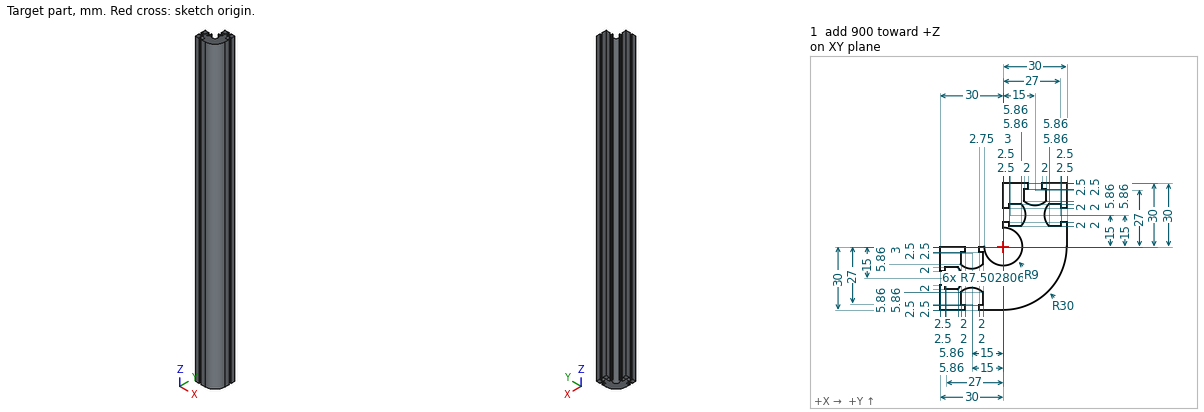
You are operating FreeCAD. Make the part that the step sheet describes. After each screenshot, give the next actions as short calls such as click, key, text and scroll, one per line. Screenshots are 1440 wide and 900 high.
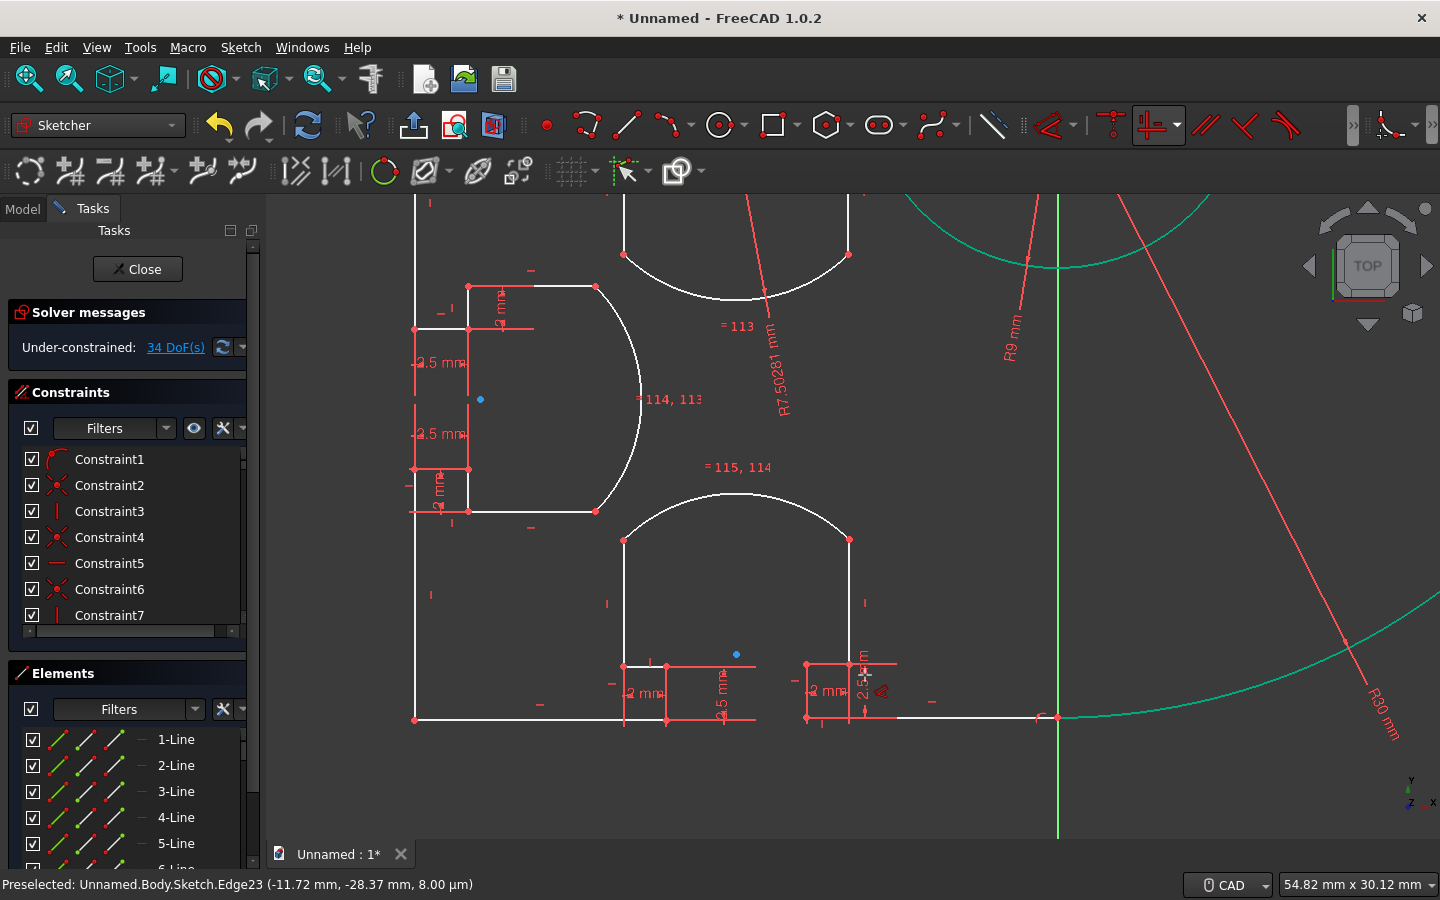
scroll(667, 707, down, 6)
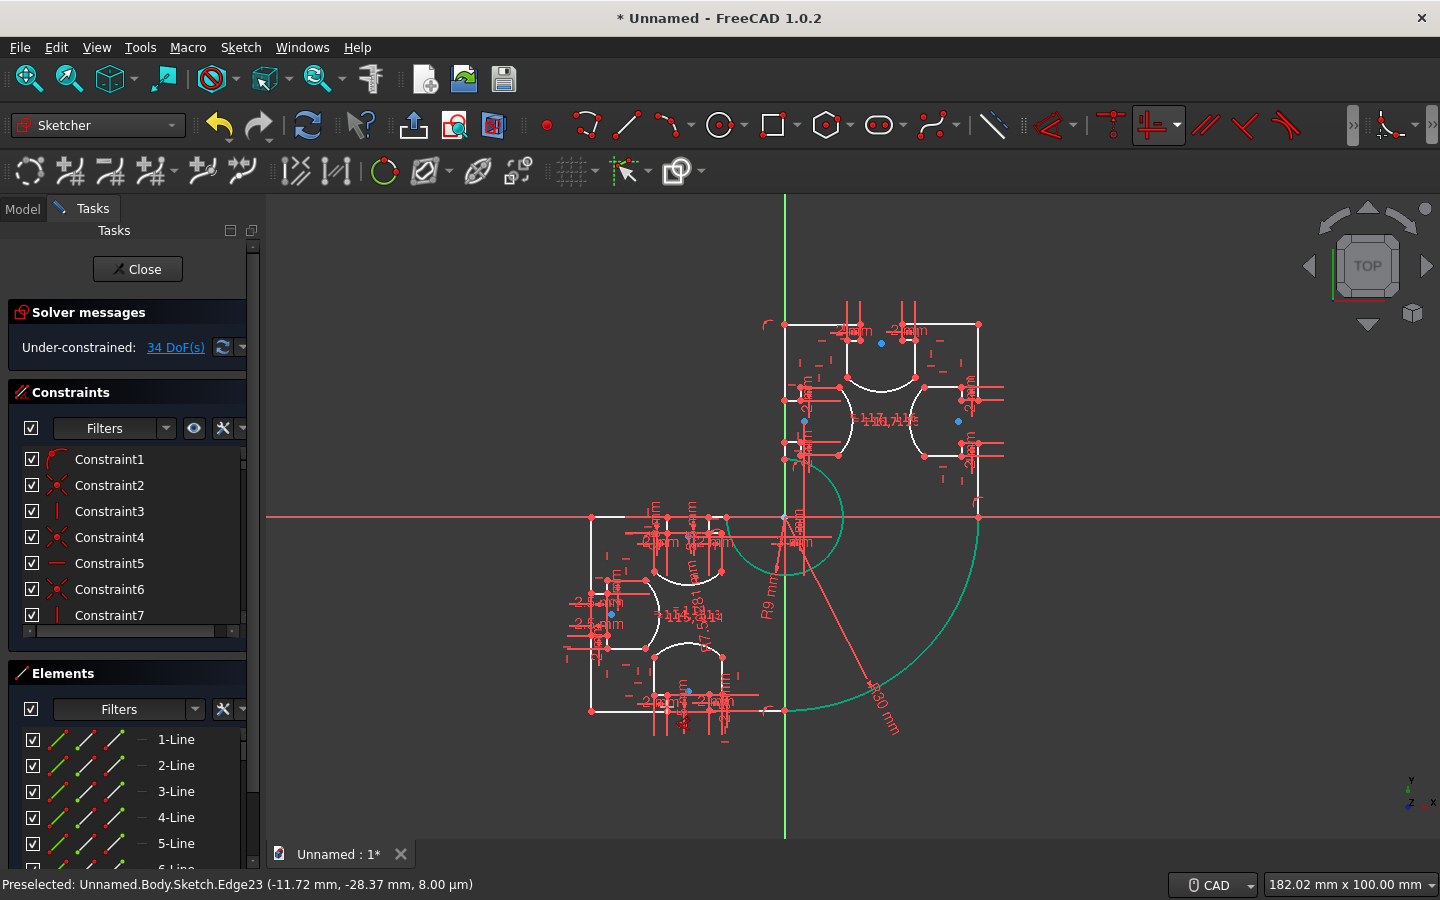
scroll(973, 443, up, 6)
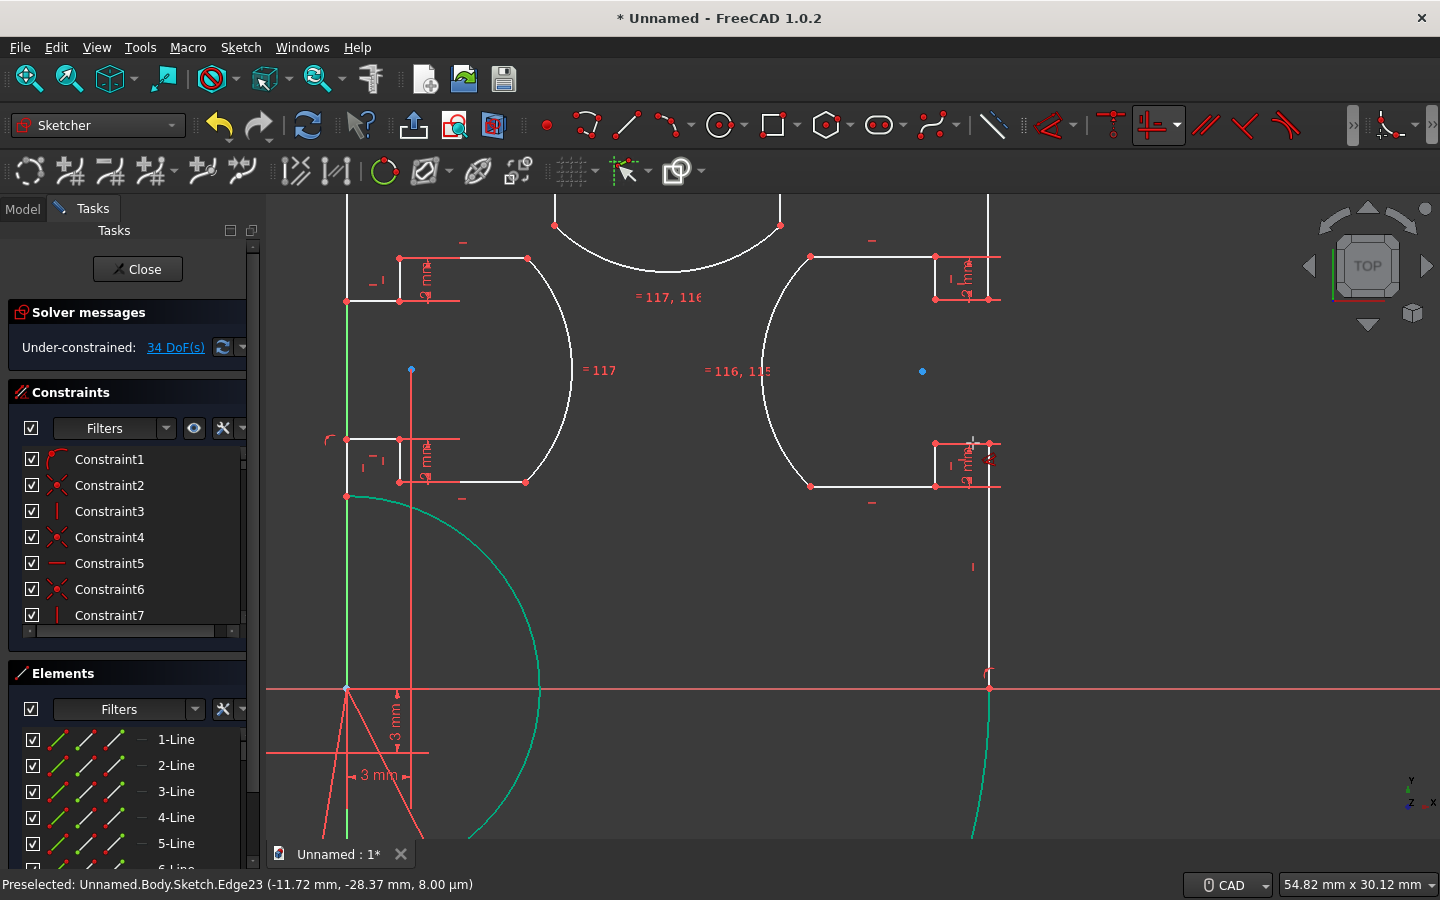
click(973, 444)
click(962, 410)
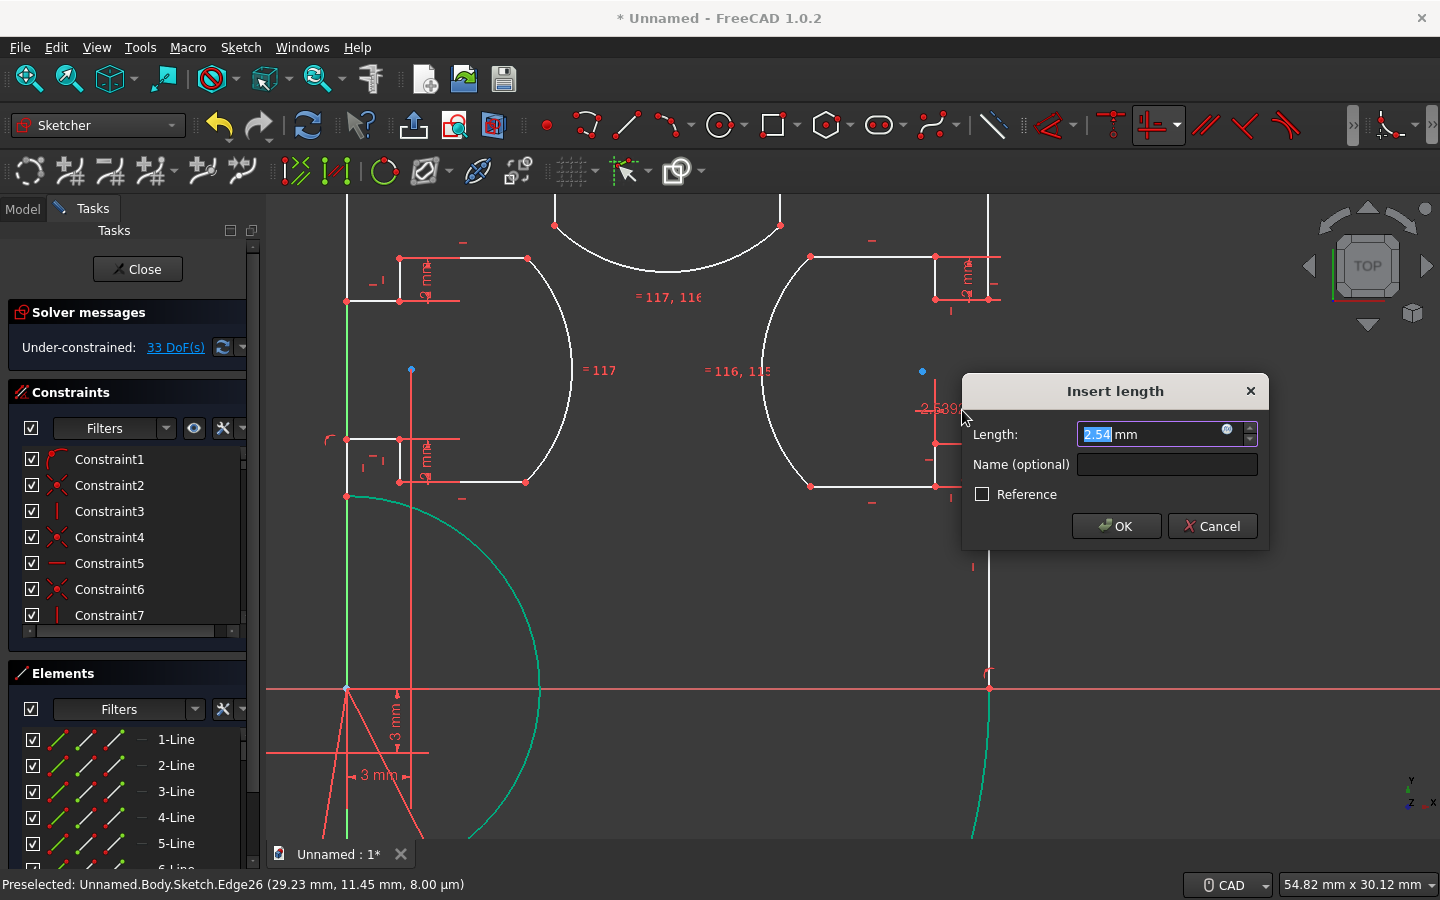
text(2.5)
key(Return)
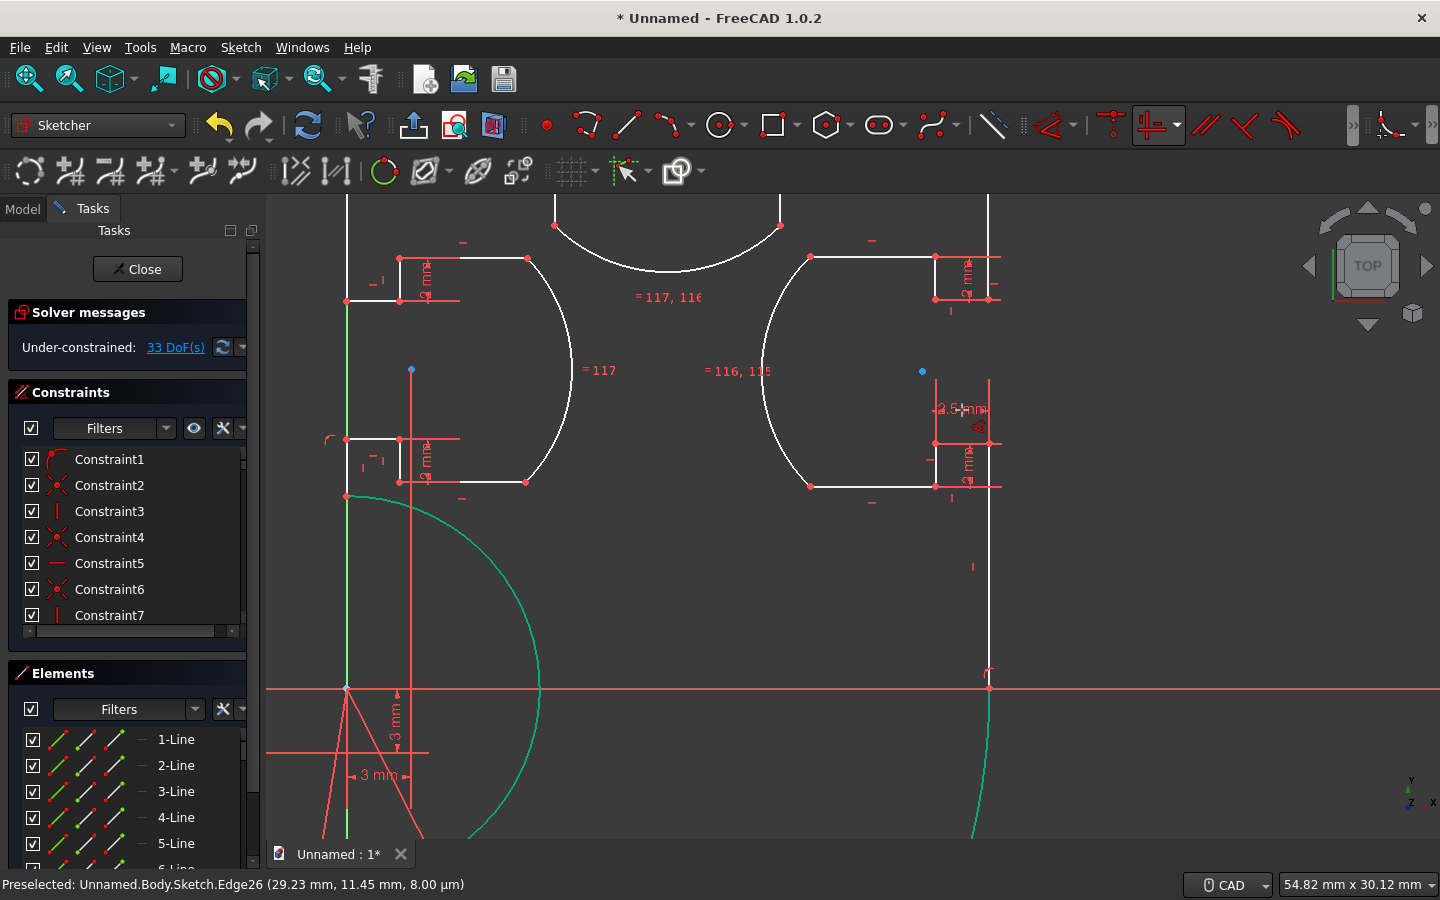
click(951, 300)
click(962, 334)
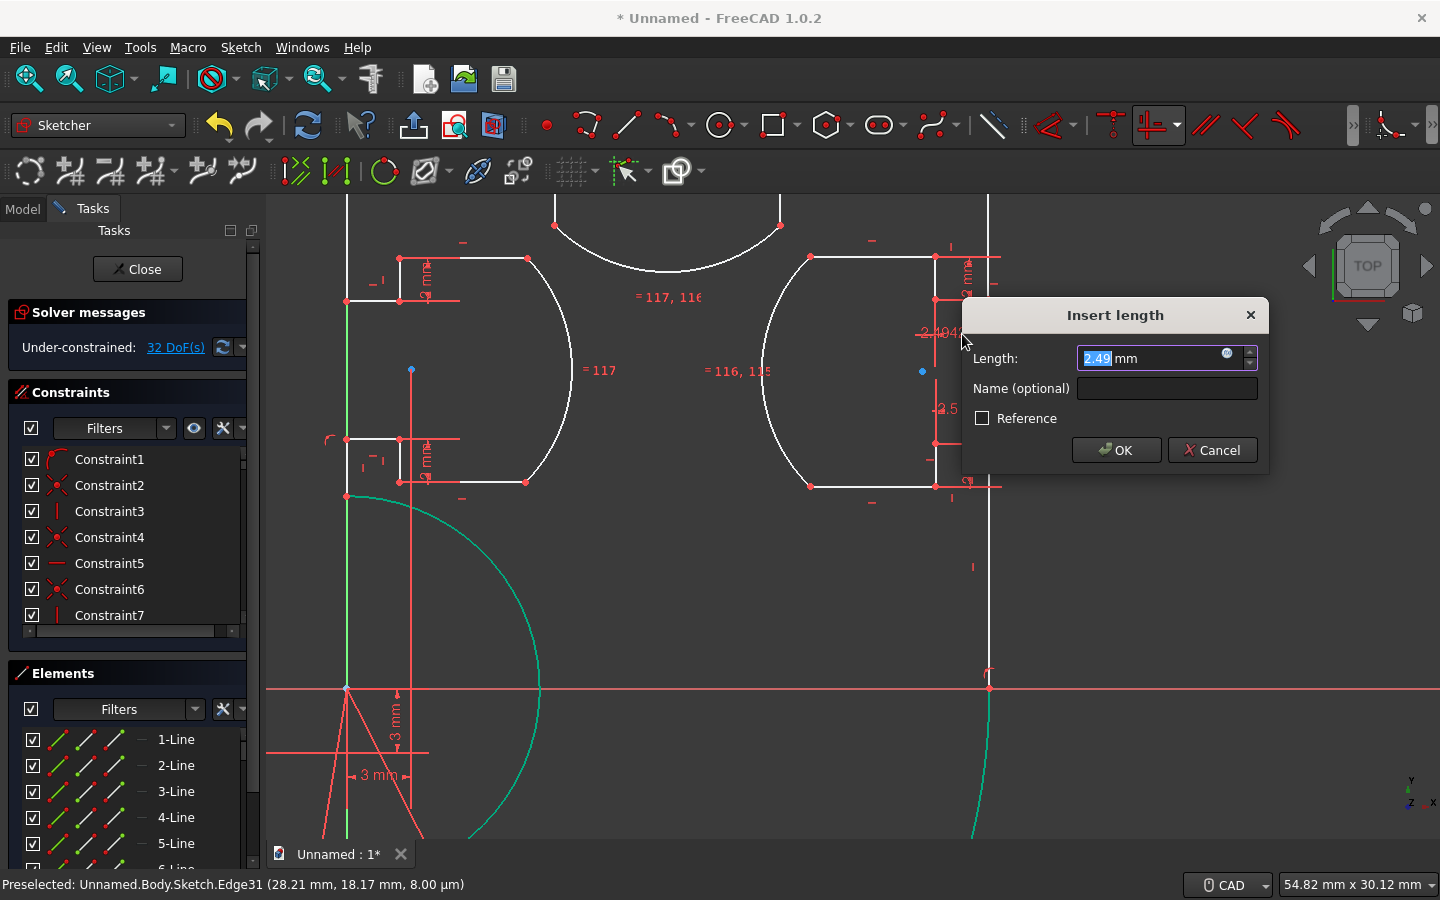
text(2.5)
key(Return)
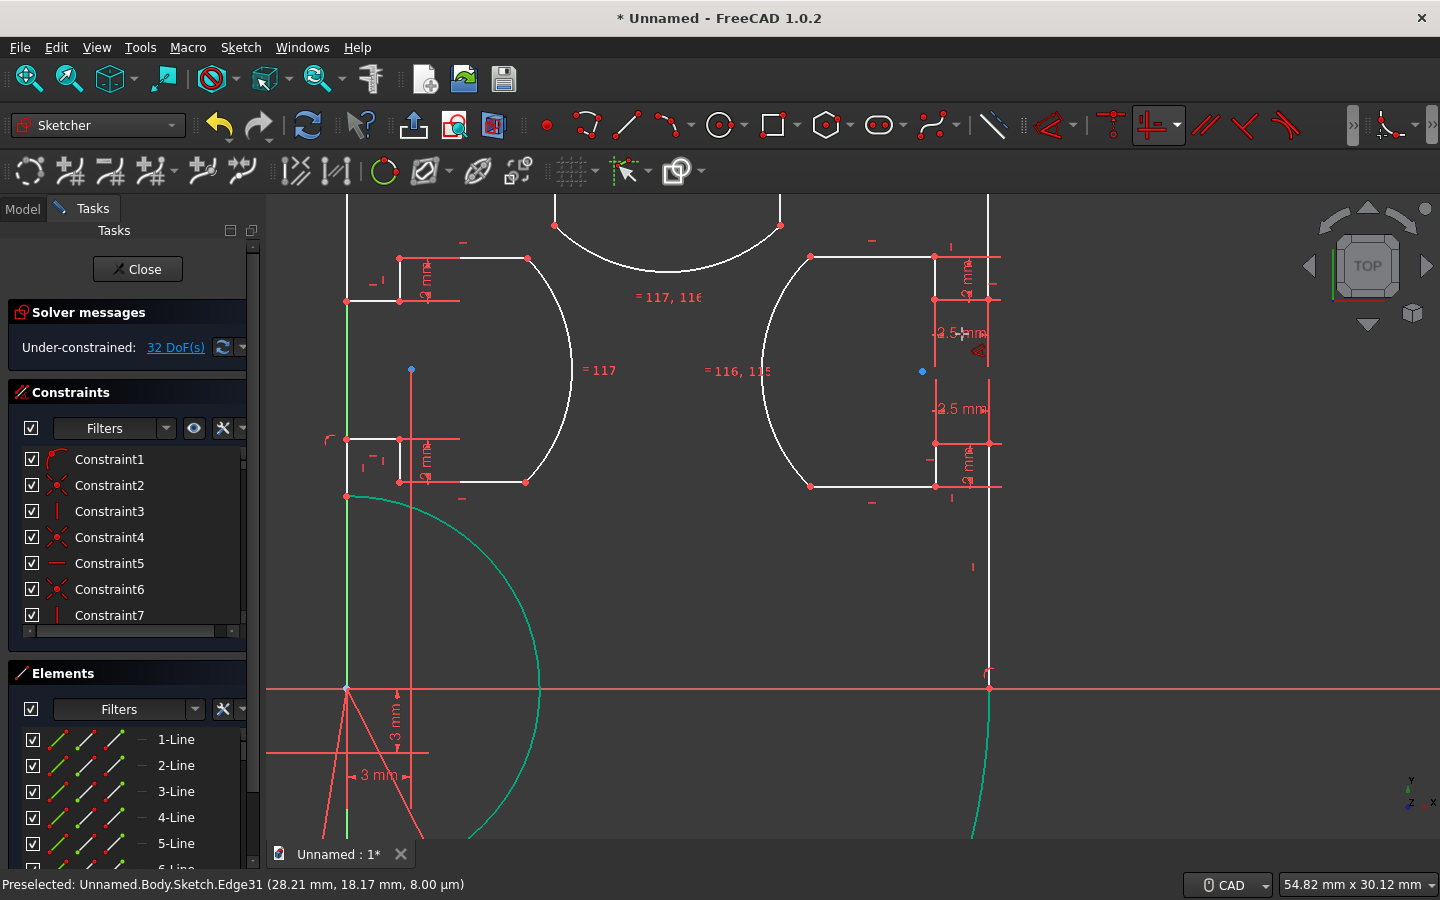
scroll(973, 442, down, 6)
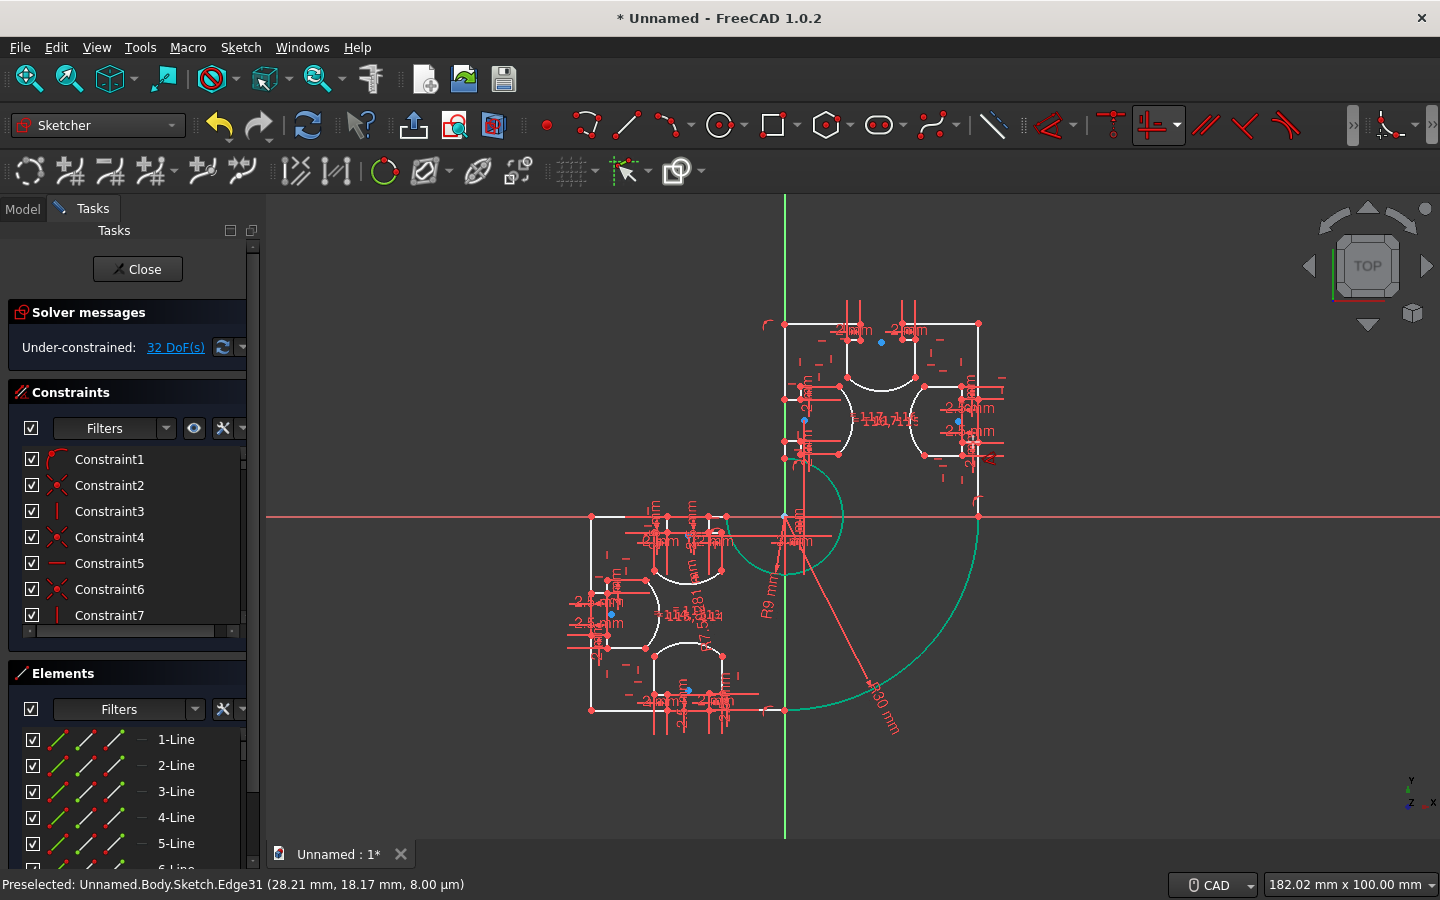
scroll(902, 329, up, 6)